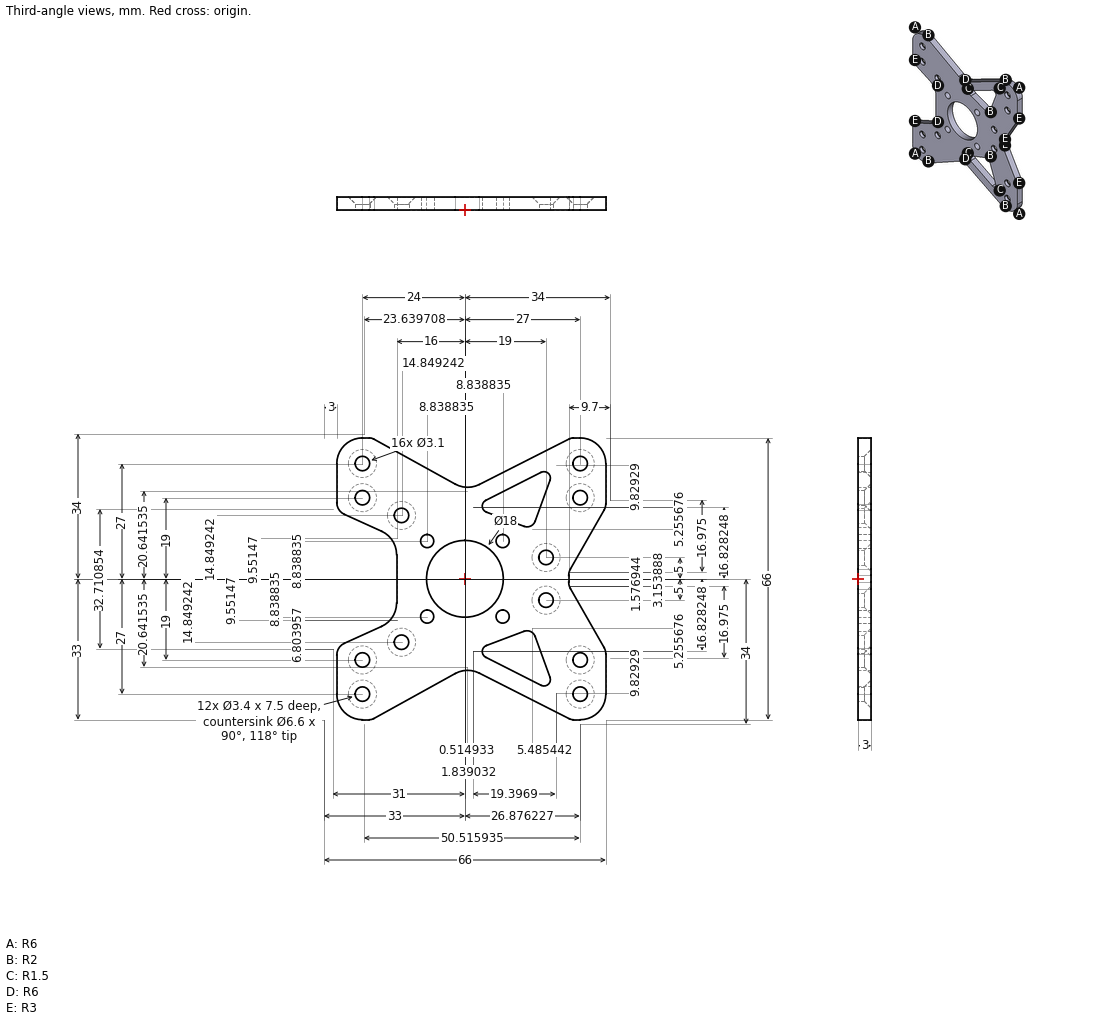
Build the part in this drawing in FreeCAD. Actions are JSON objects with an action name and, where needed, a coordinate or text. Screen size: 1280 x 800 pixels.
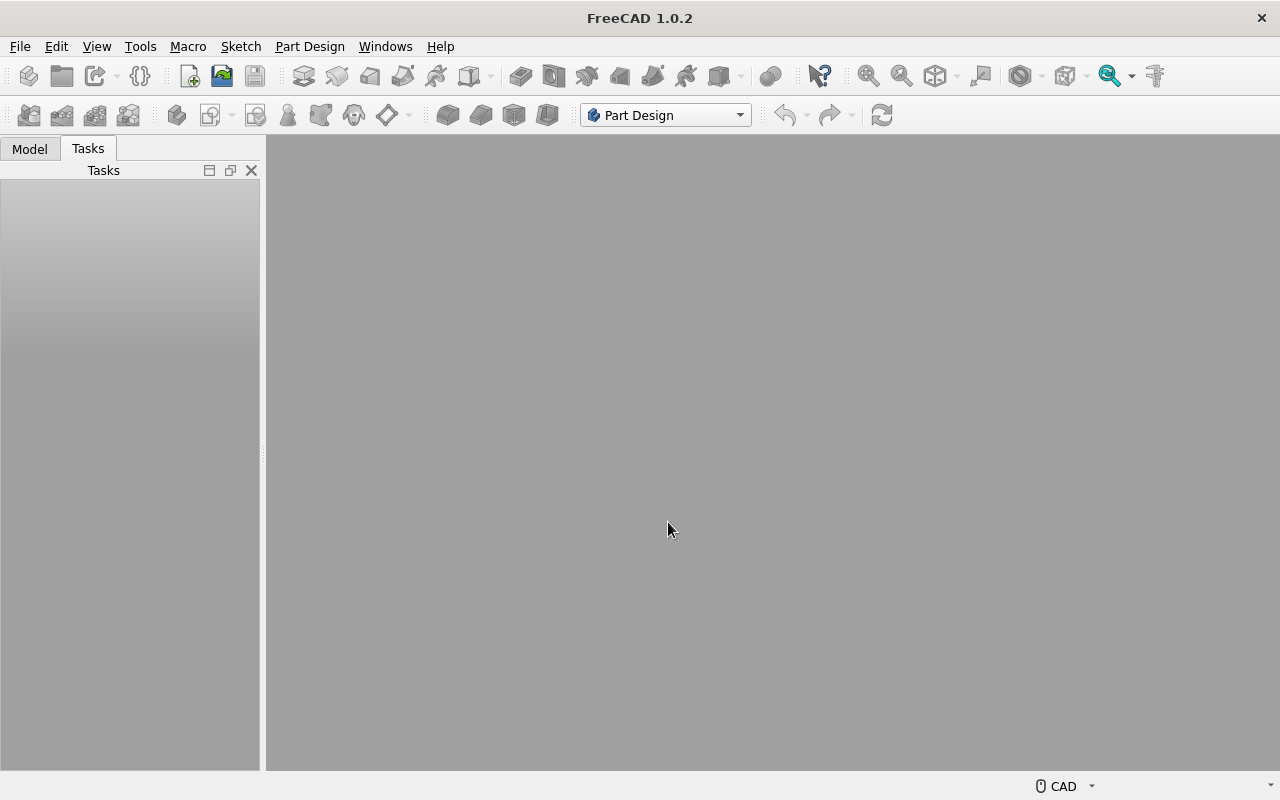
{"action": "left_click", "coordinate": [189, 76]}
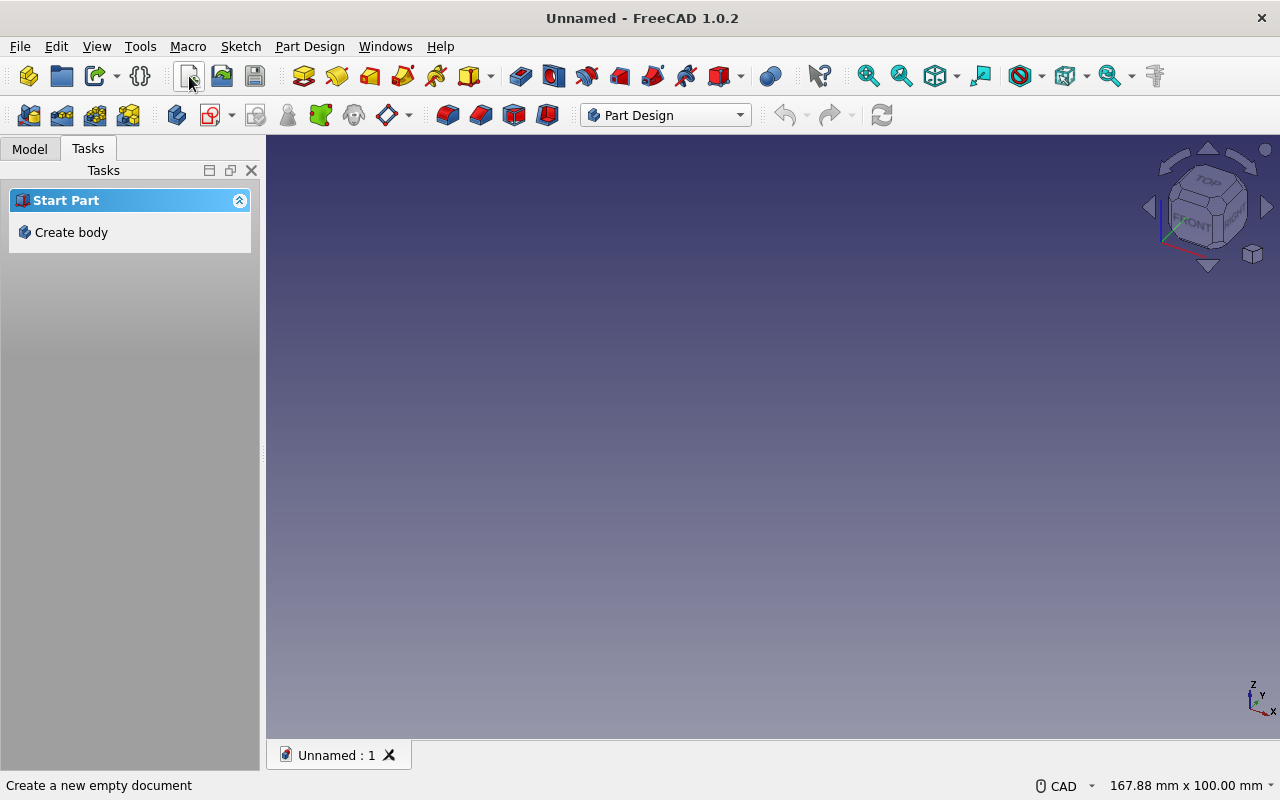
{"action": "left_click", "coordinate": [210, 116]}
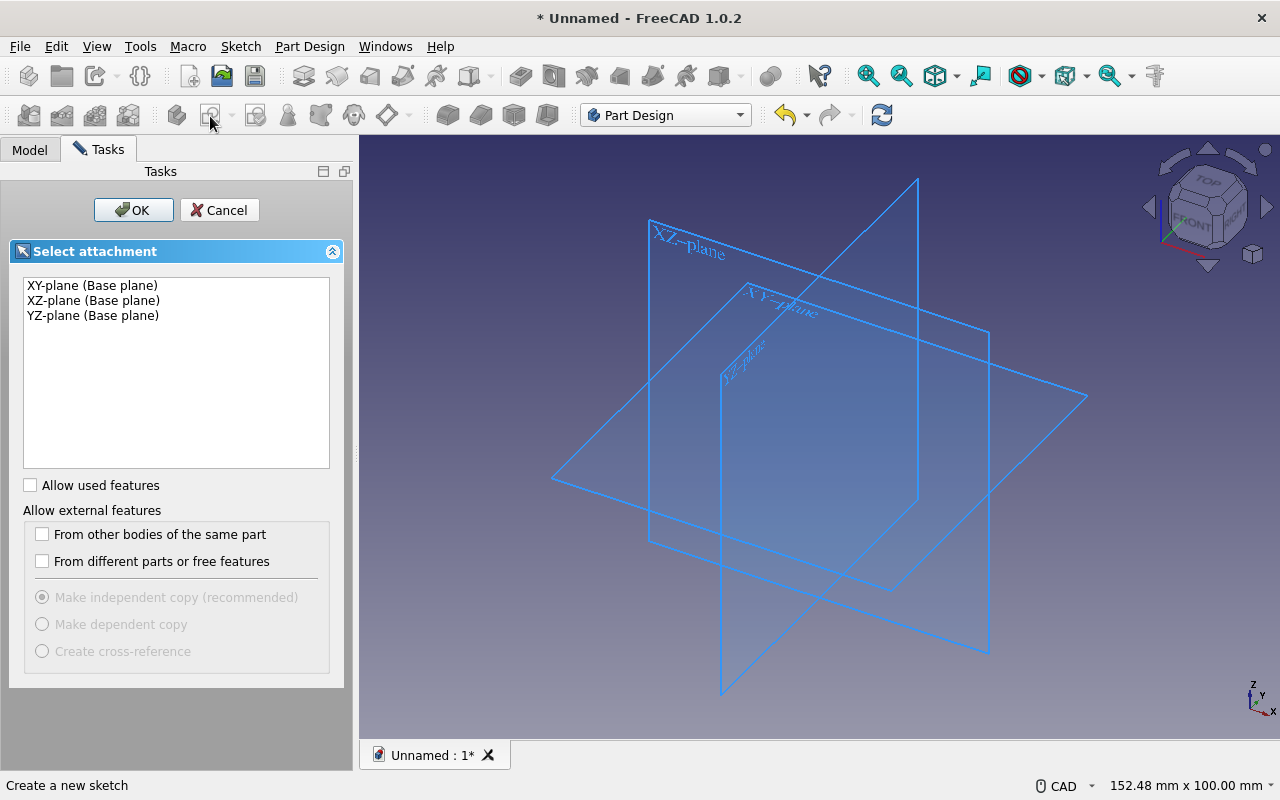
{"action": "left_click", "coordinate": [84, 300]}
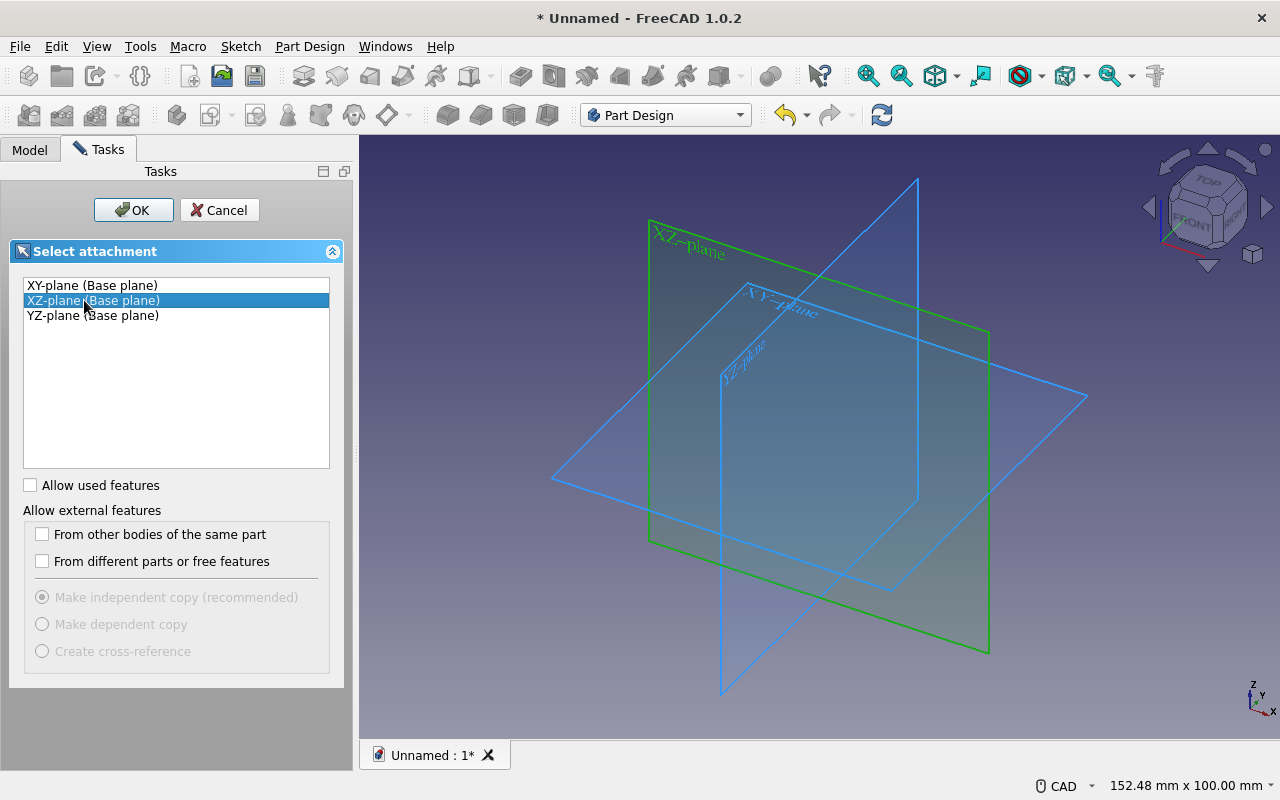
{"action": "left_click", "coordinate": [134, 210]}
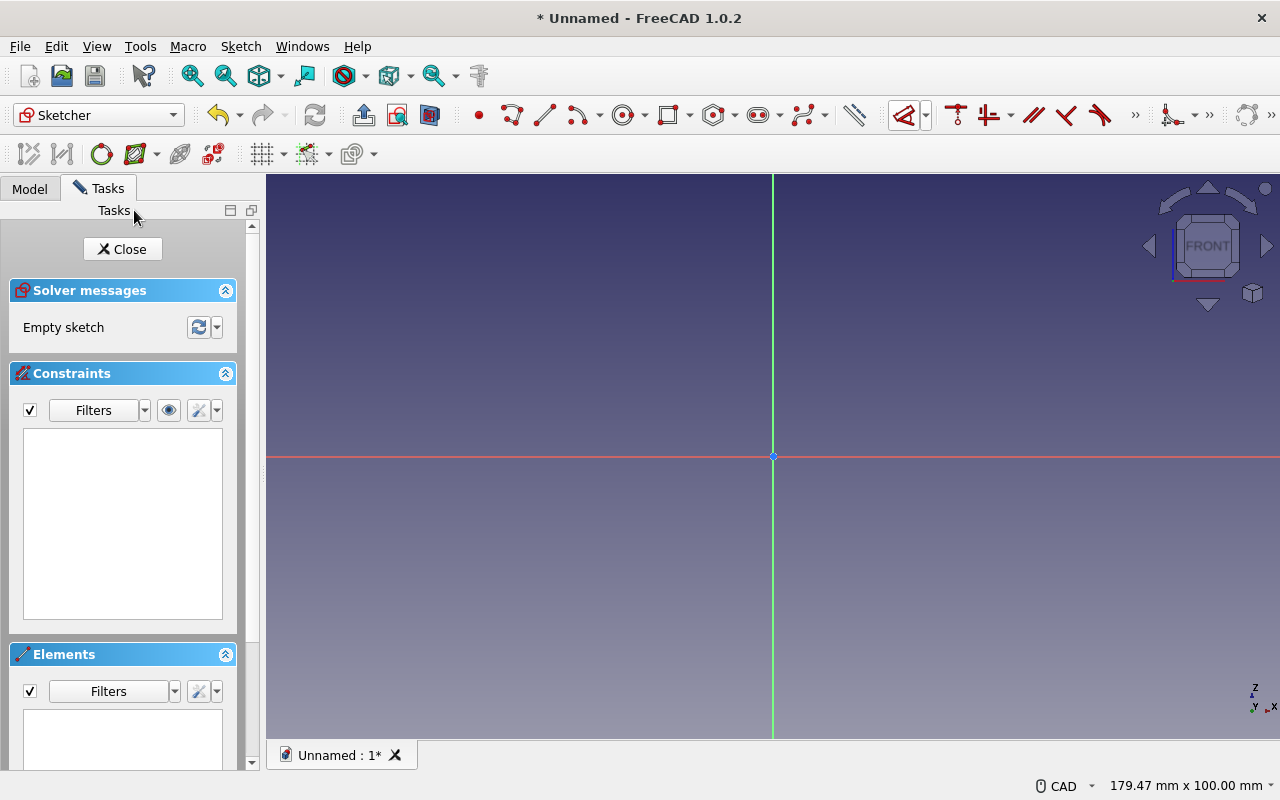
{"action": "key", "text": "g v"}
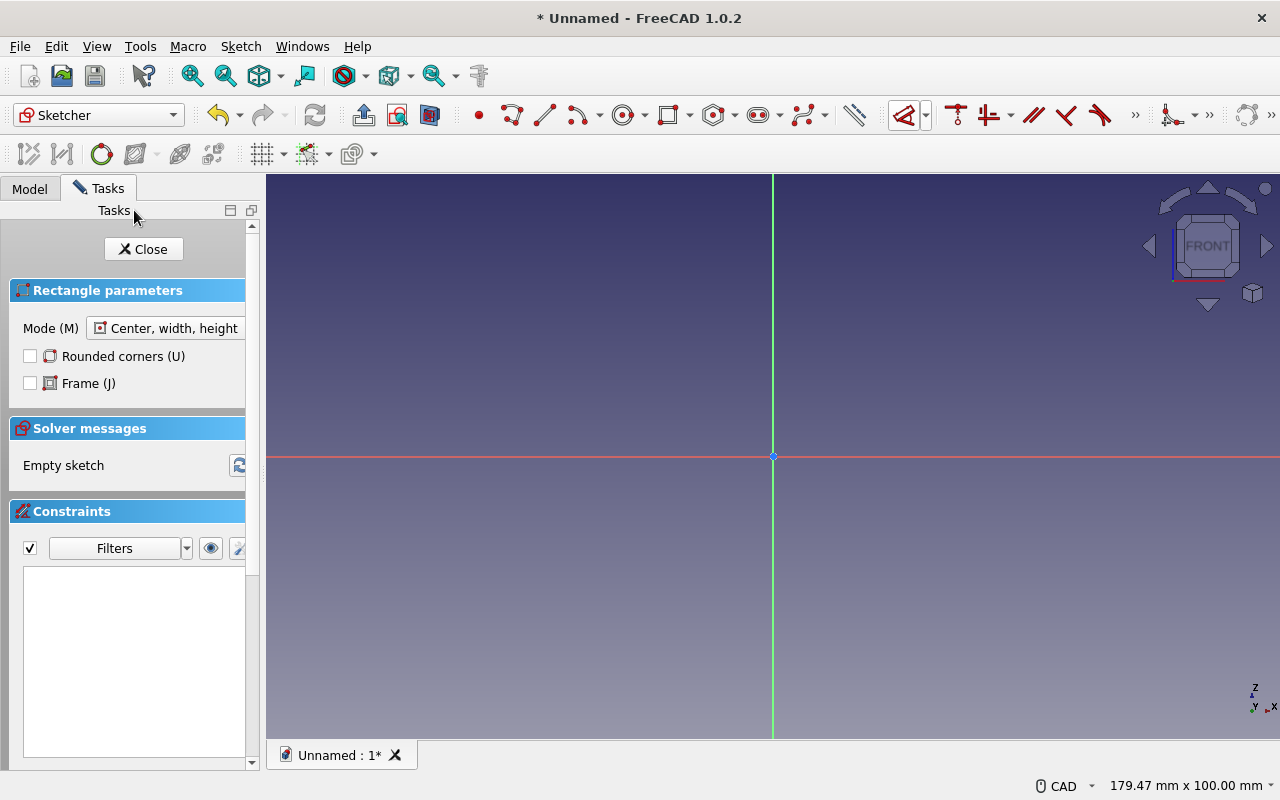
{"action": "left_click", "coordinate": [773, 456]}
{"action": "mouse_move", "coordinate": [959, 270]}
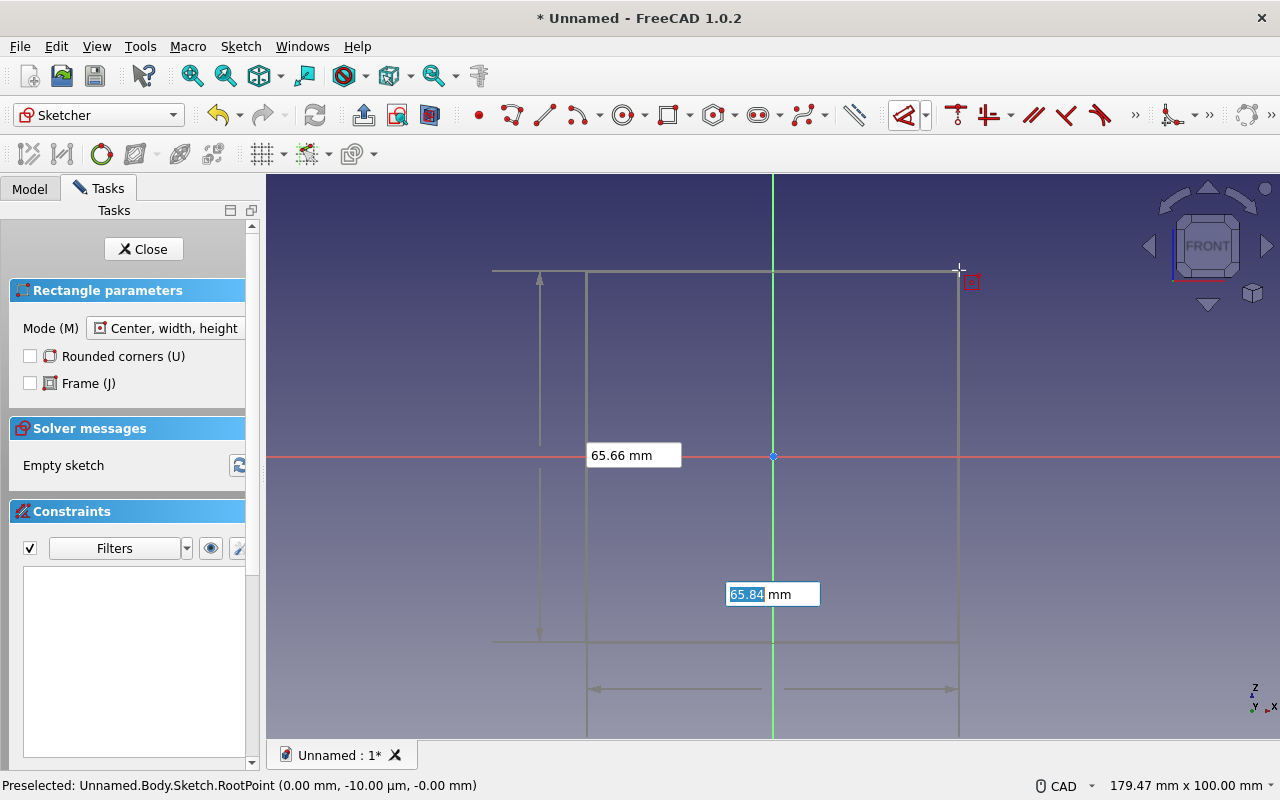
{"action": "type", "text": "66"}
{"action": "key", "text": "Tab"}
{"action": "type", "text": "66"}
{"action": "key", "text": "Return"}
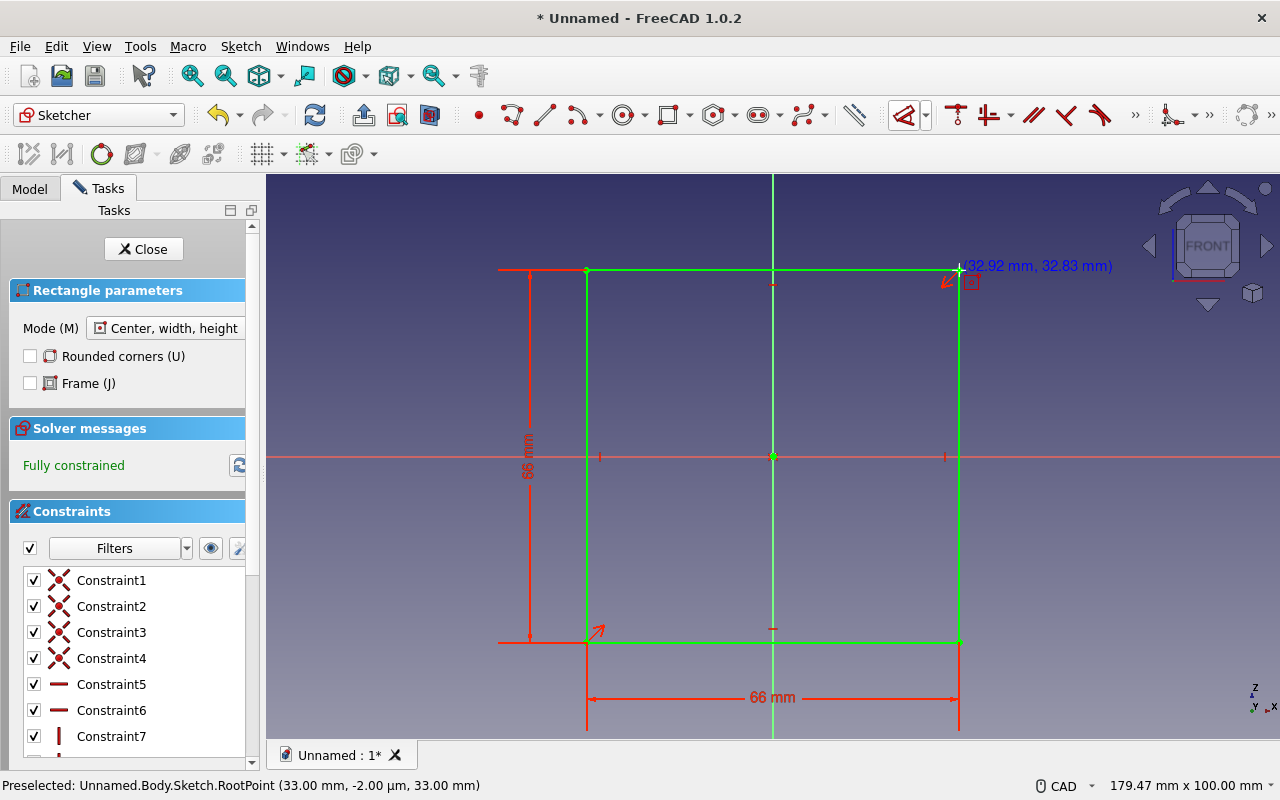
{"action": "left_click", "coordinate": [622, 116]}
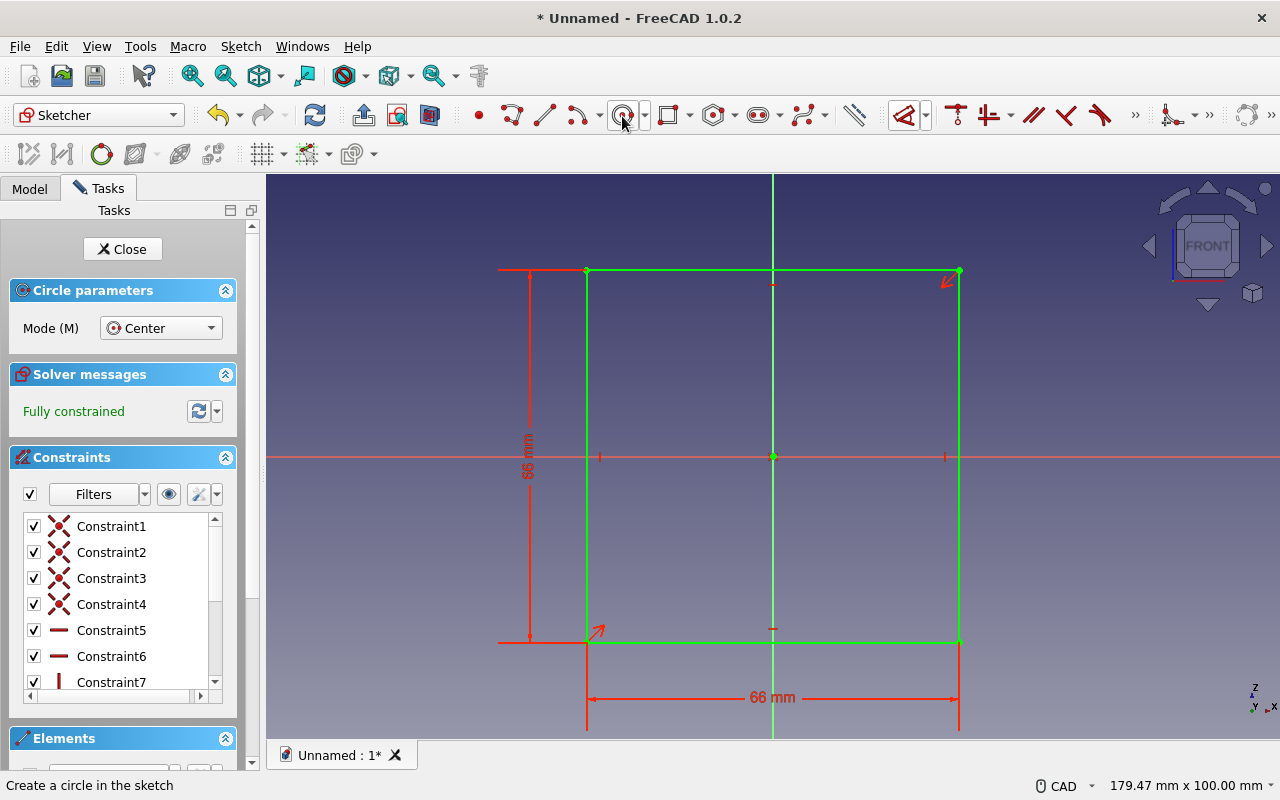
{"action": "scroll", "coordinate": [637, 304], "scroll_direction": "up", "scroll_amount": 5}